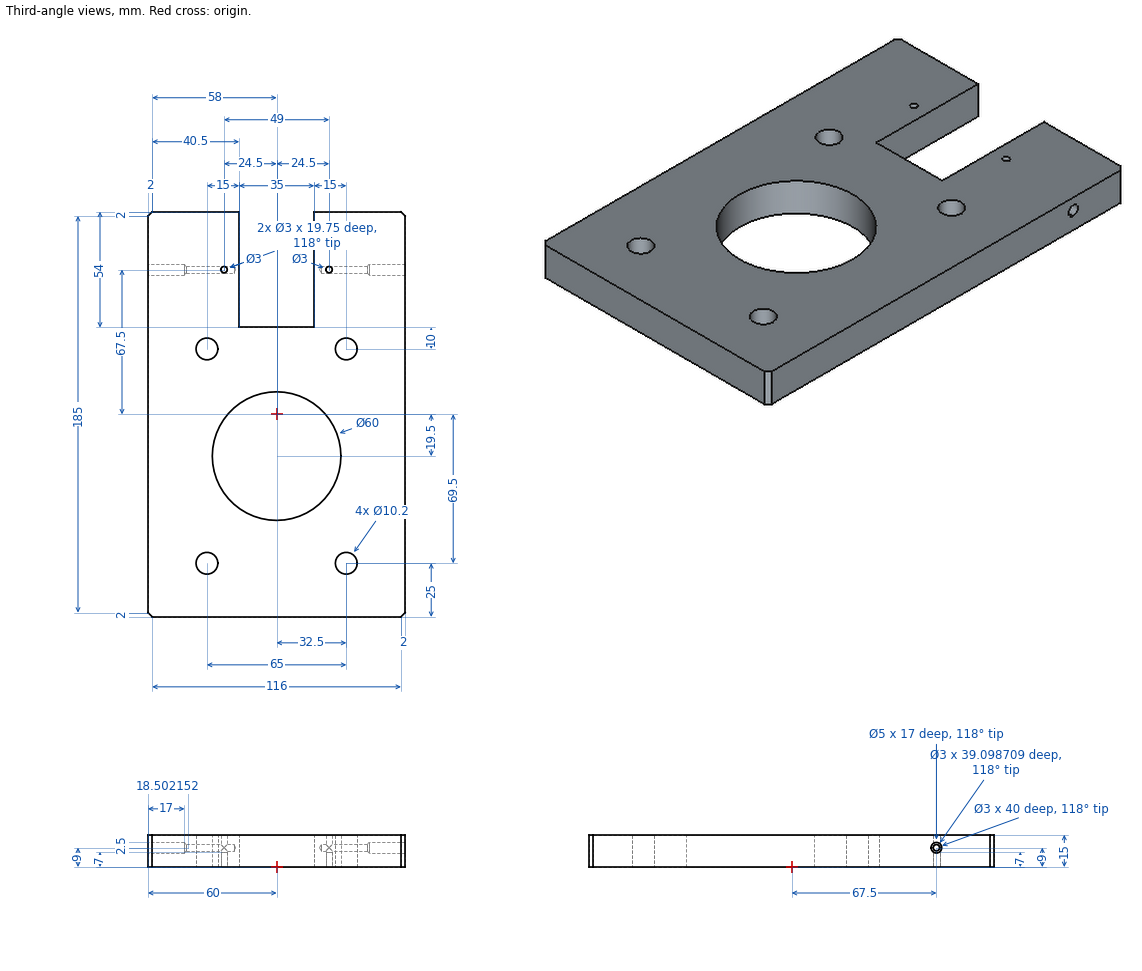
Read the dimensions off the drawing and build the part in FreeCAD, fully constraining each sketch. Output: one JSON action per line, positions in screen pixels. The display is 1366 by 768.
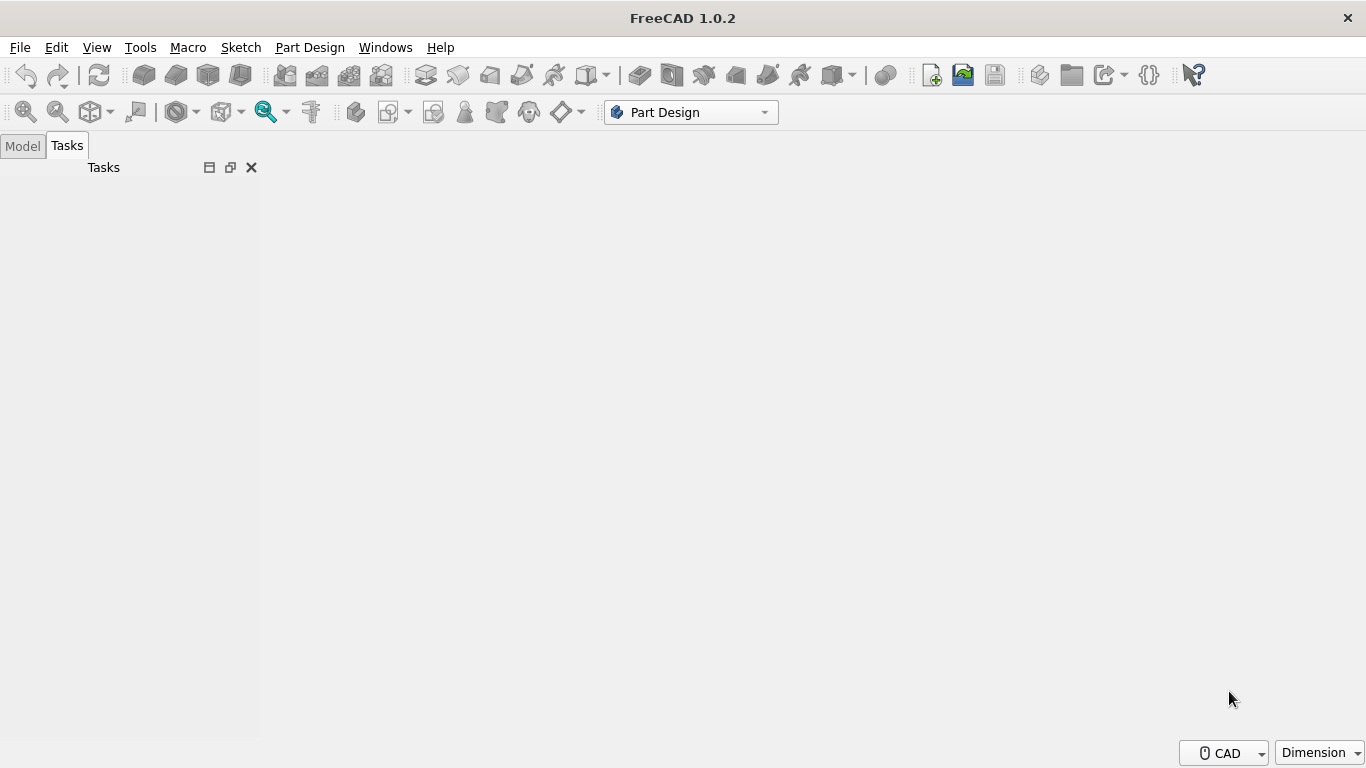
{"action": "key", "text": "ctrl+n"}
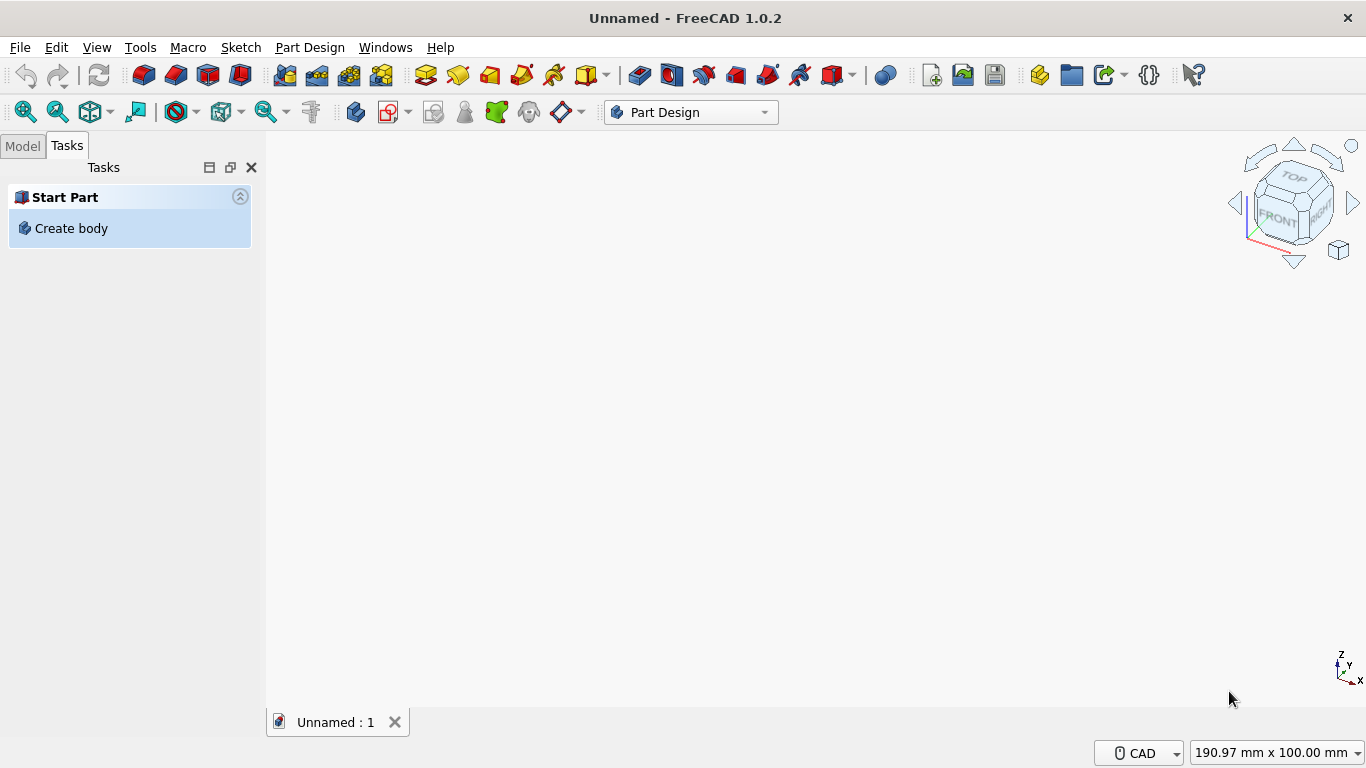
{"action": "left_click", "coordinate": [388, 112]}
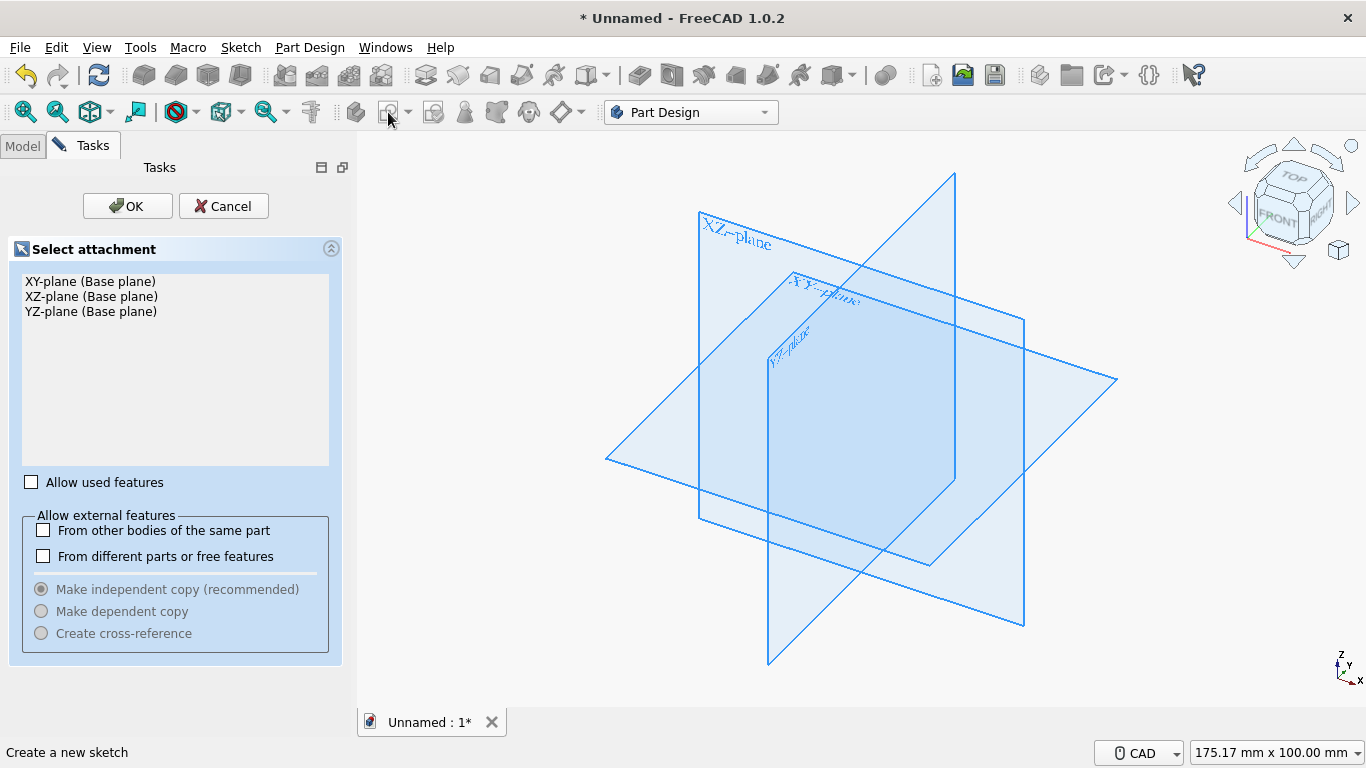
{"action": "left_click", "coordinate": [82, 282]}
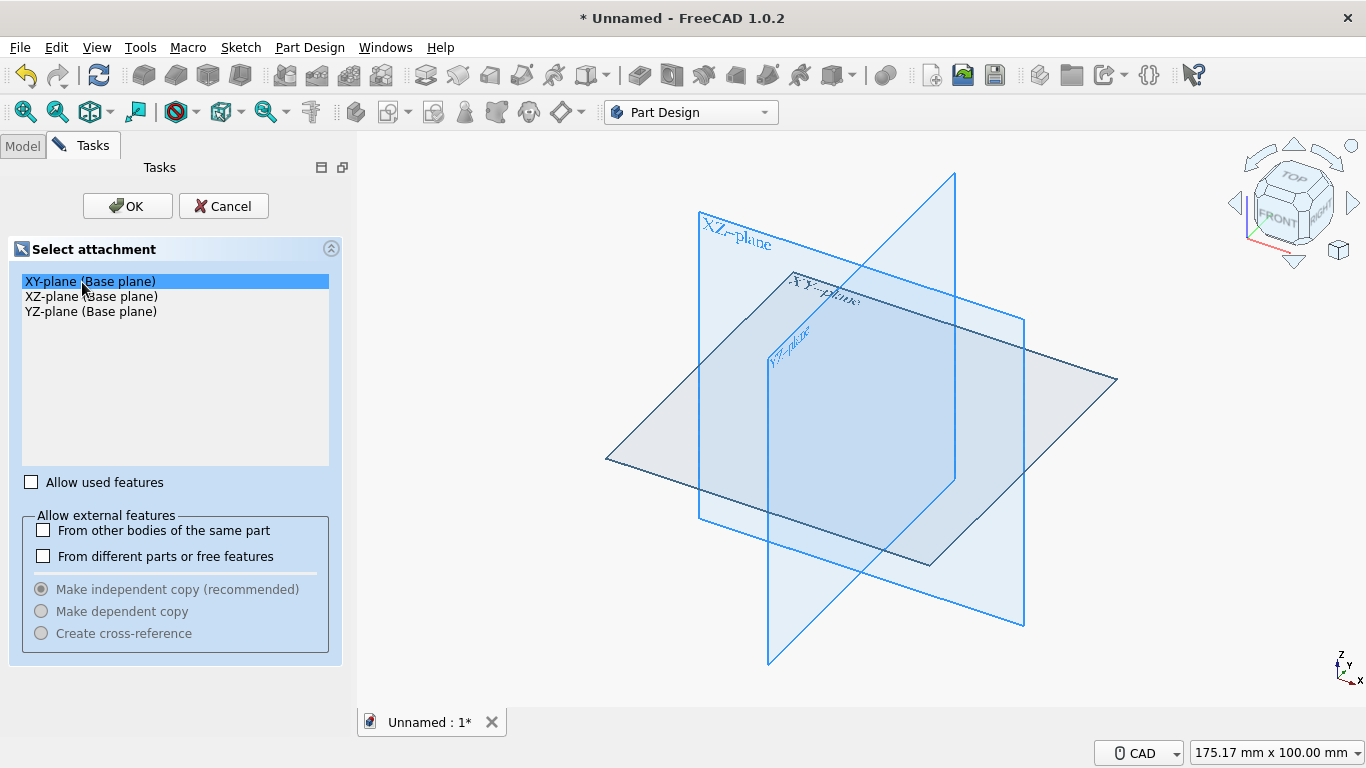
{"action": "left_click", "coordinate": [128, 206]}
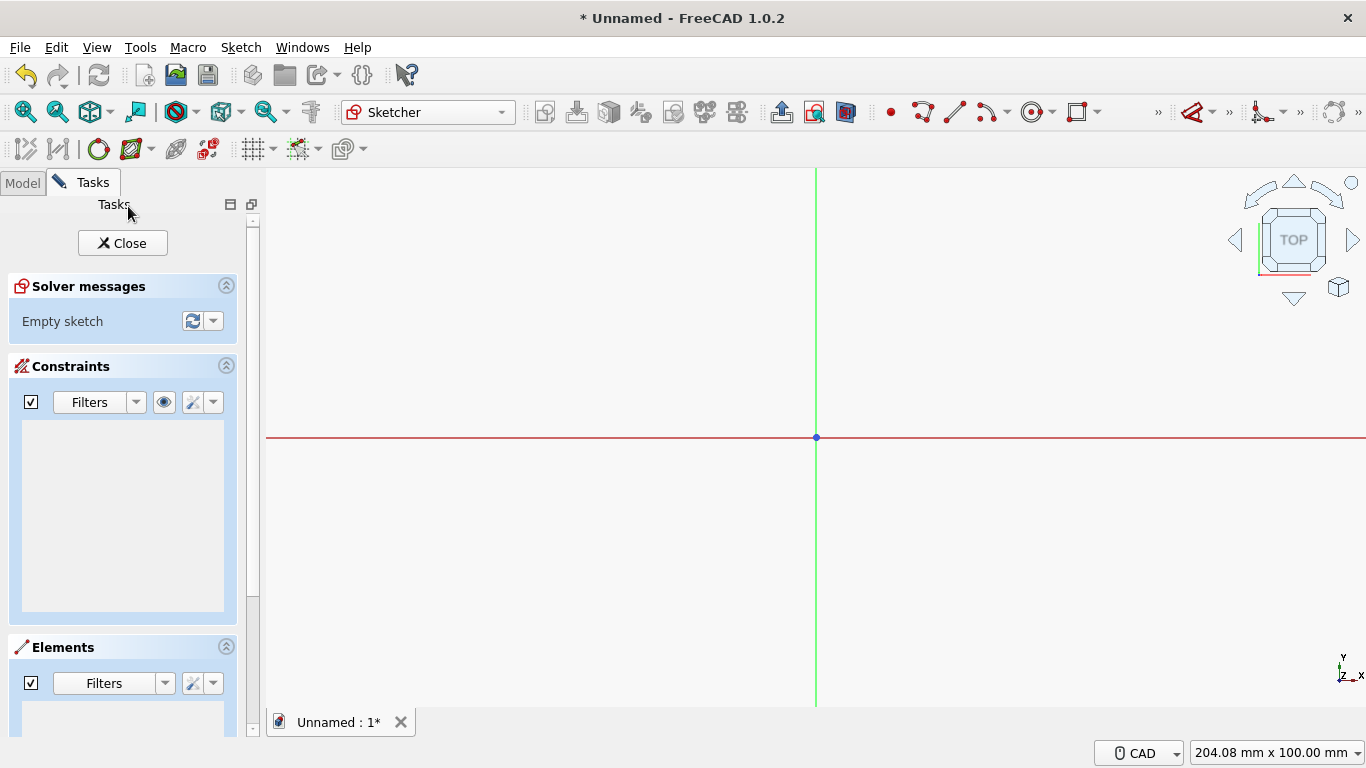
{"action": "scroll", "coordinate": [708, 438], "scroll_direction": "down", "scroll_amount": 5}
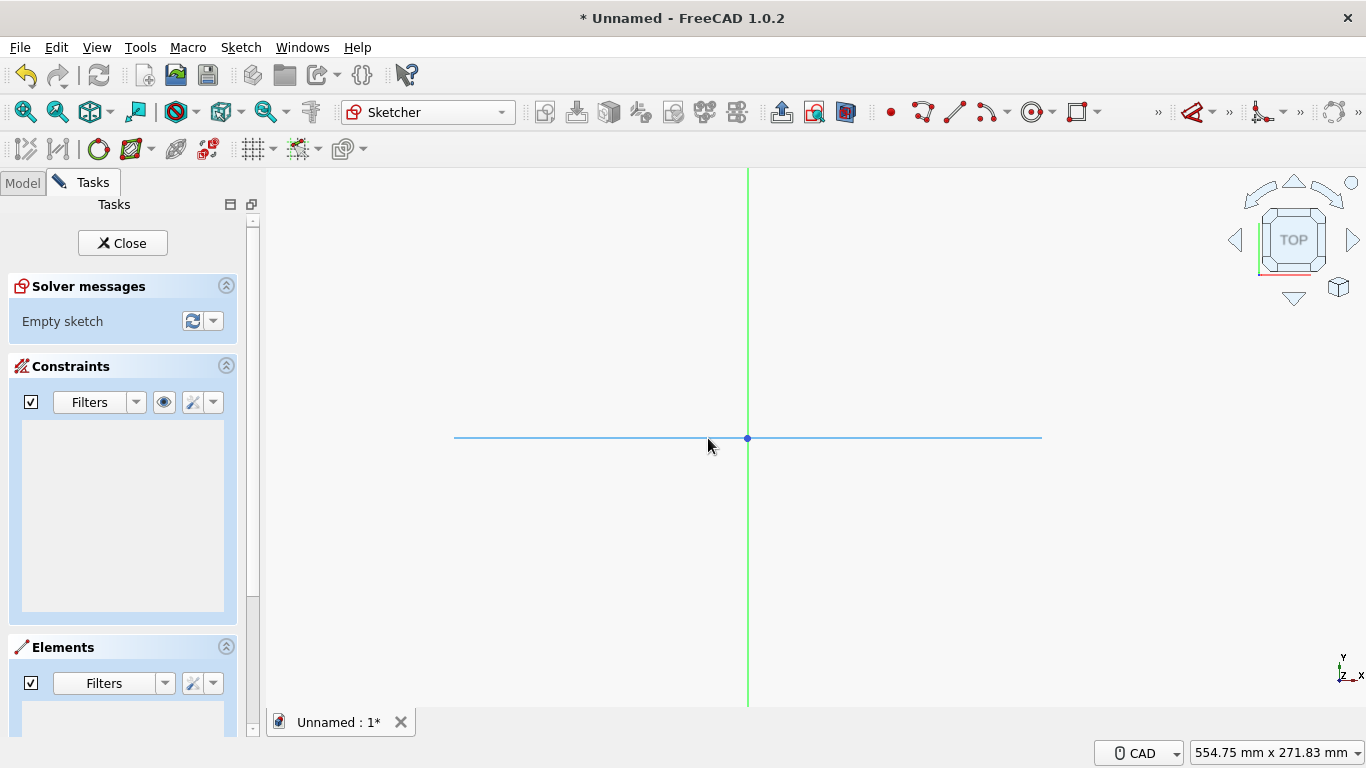
{"action": "key", "text": "g m"}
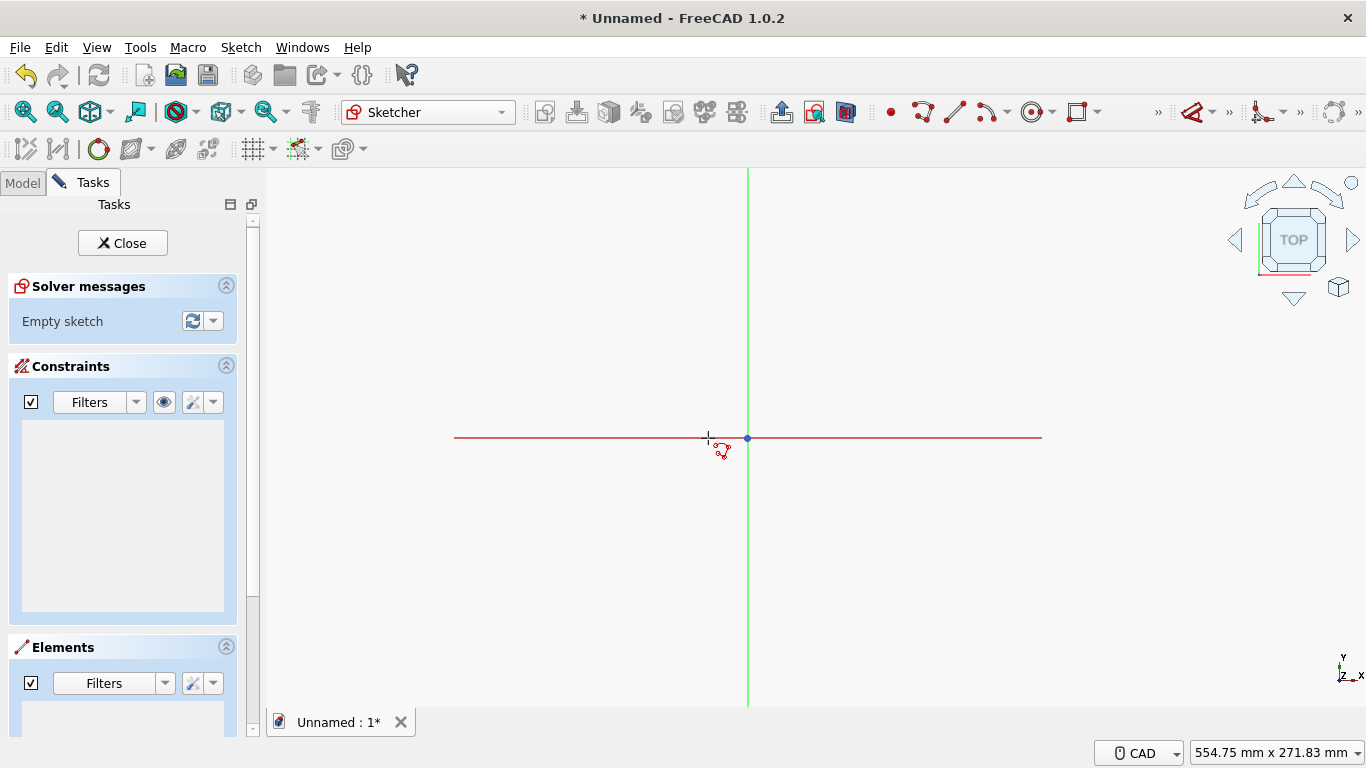
{"action": "left_click", "coordinate": [783, 358]}
{"action": "left_click", "coordinate": [713, 358]}
{"action": "left_click", "coordinate": [713, 251]}
{"action": "left_click", "coordinate": [633, 251]}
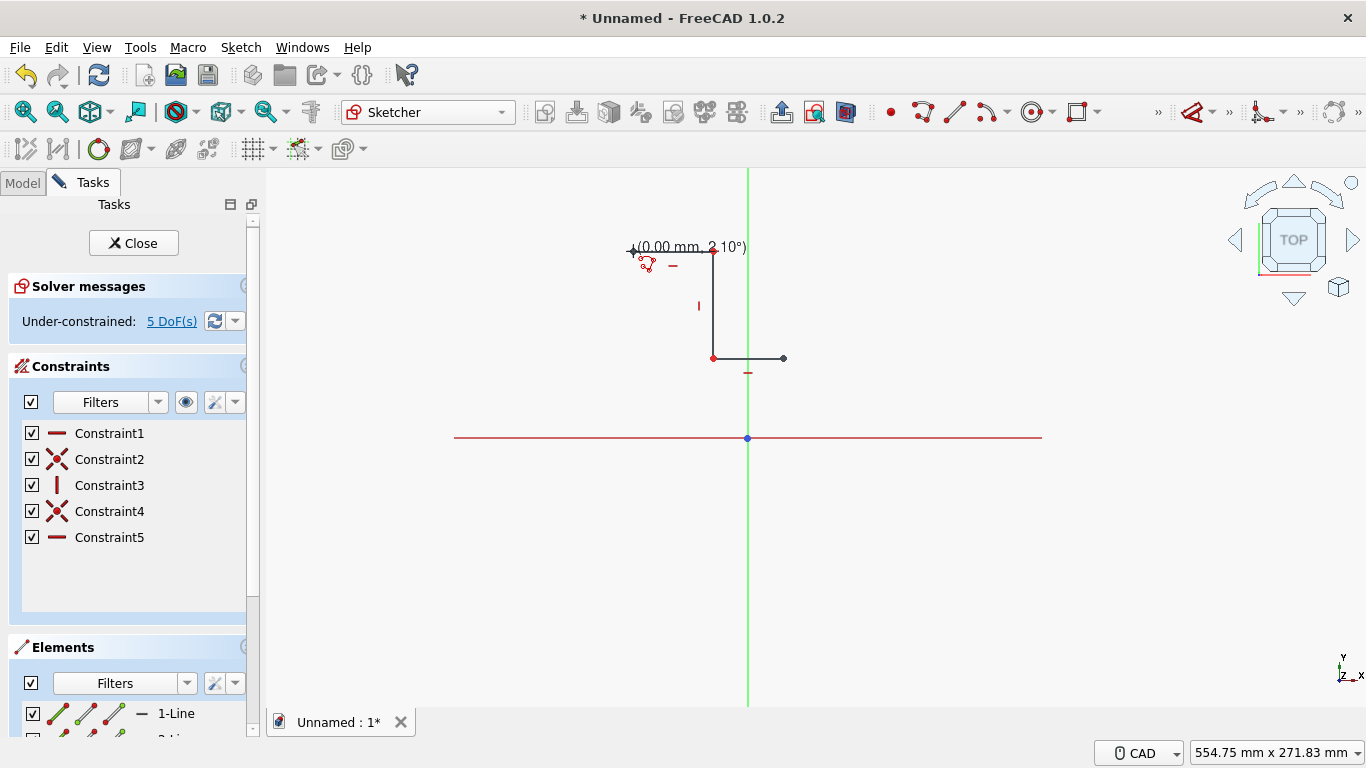
{"action": "scroll", "coordinate": [629, 255], "scroll_direction": "up", "scroll_amount": 6}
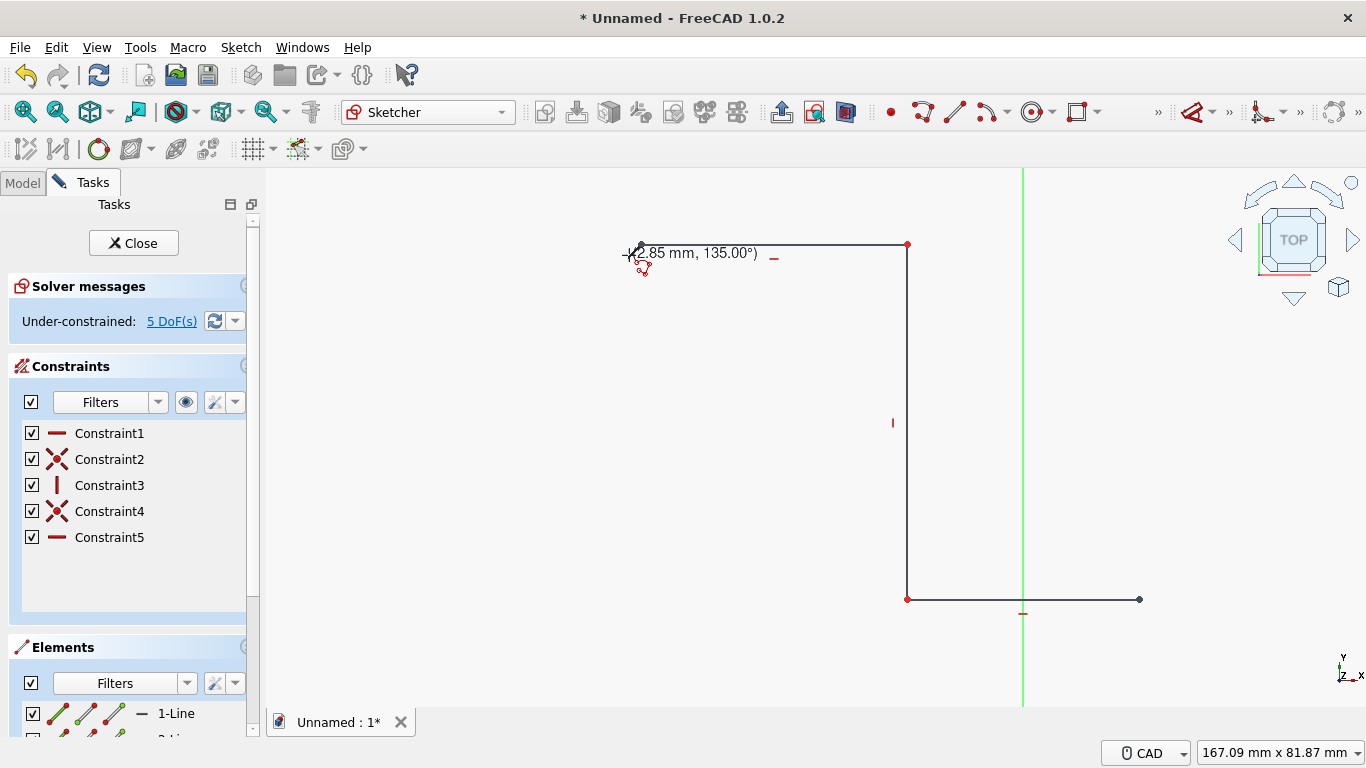
{"action": "left_click", "coordinate": [628, 254]}